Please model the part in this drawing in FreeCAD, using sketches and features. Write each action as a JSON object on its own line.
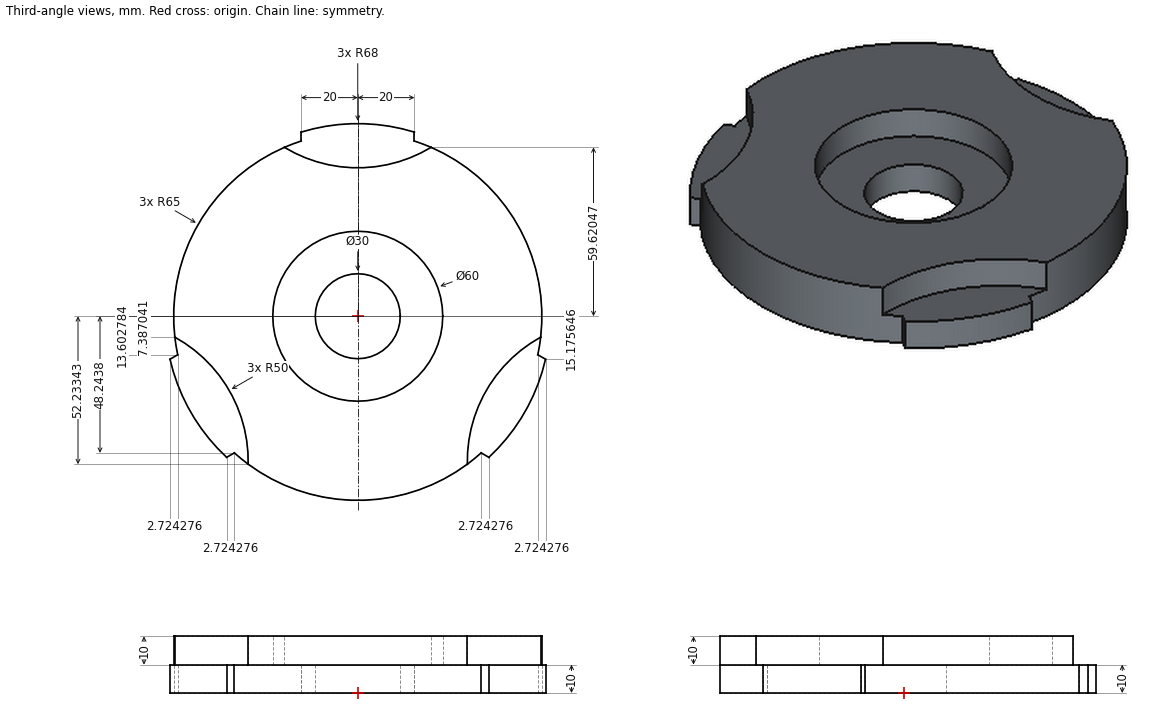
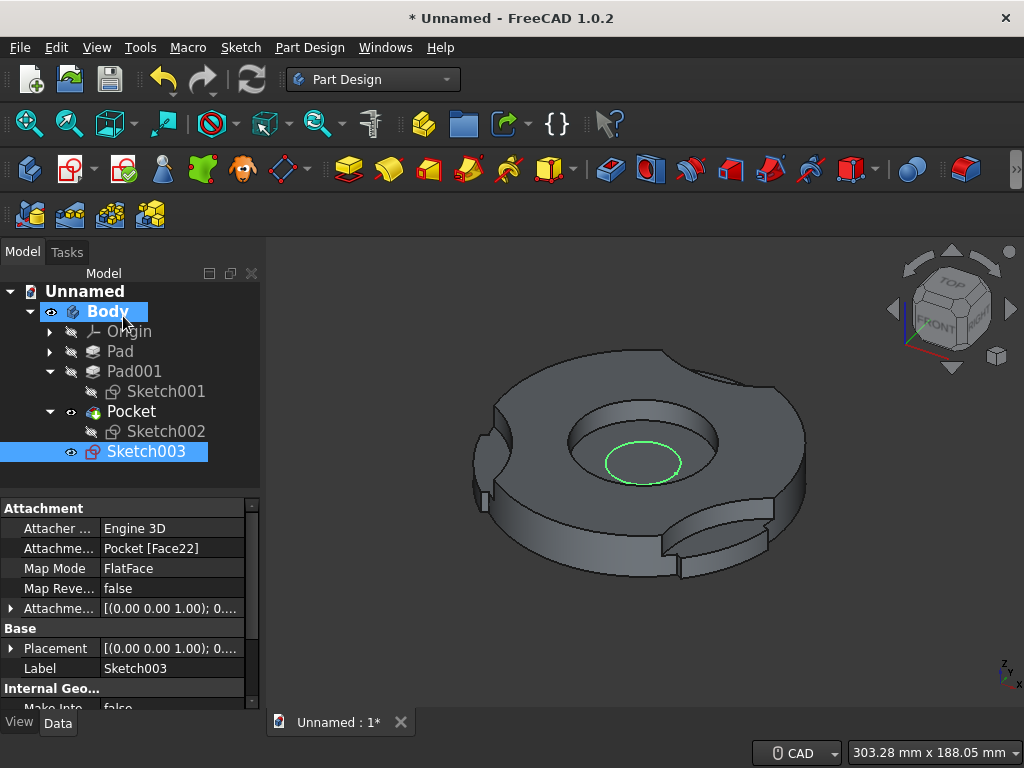
{"action": "left_click", "coordinate": [612, 170]}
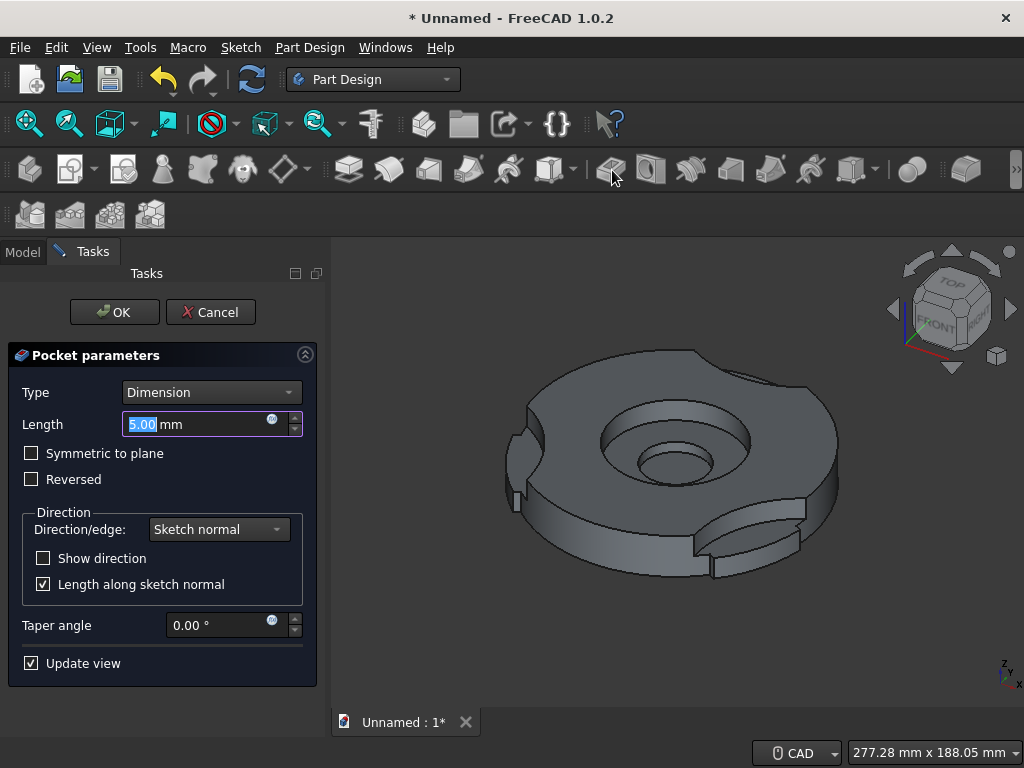
{"action": "type", "text": "10"}
{"action": "key", "text": "Tab"}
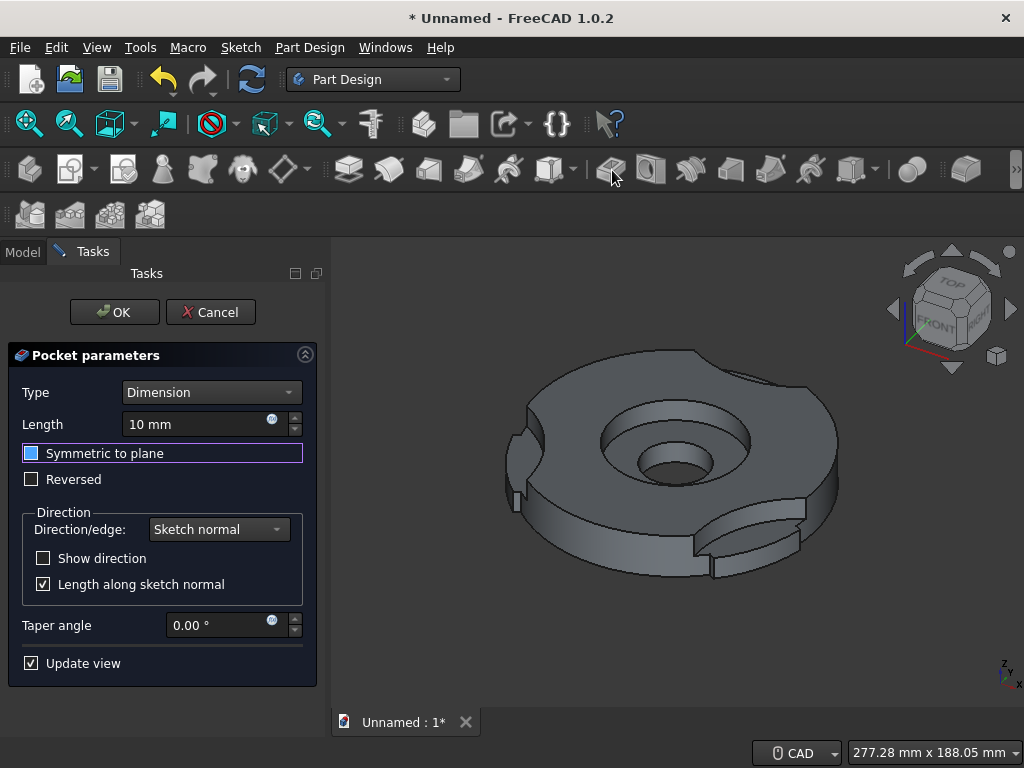
{"action": "left_click", "coordinate": [115, 312]}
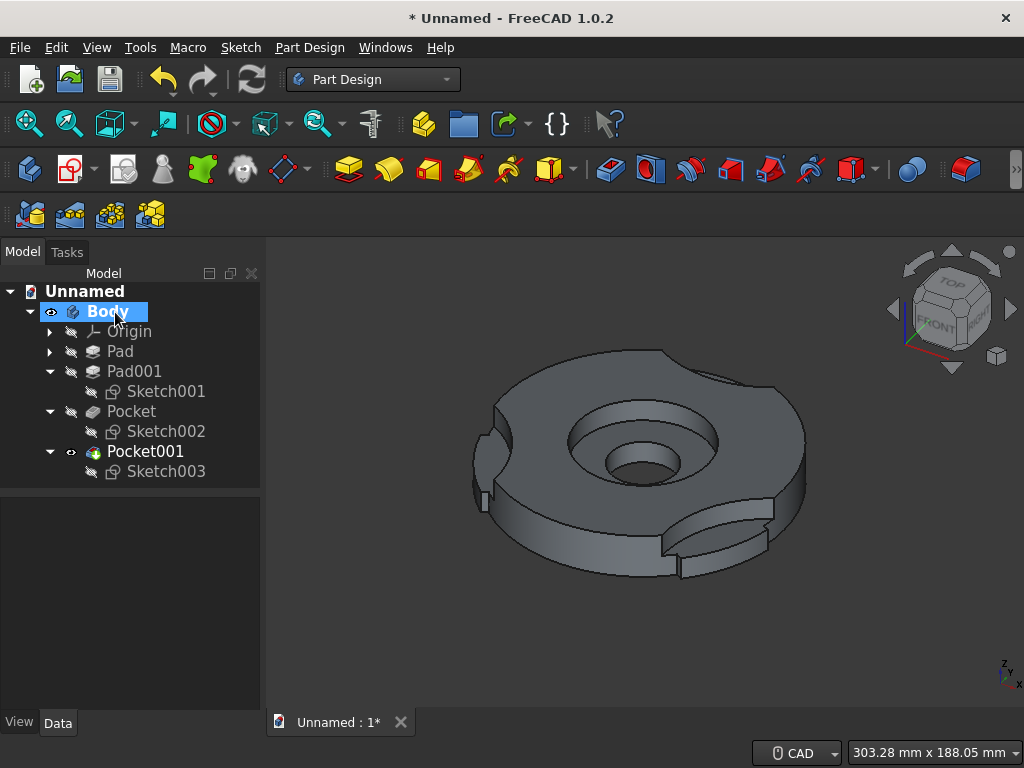
{"action": "key", "text": "0"}